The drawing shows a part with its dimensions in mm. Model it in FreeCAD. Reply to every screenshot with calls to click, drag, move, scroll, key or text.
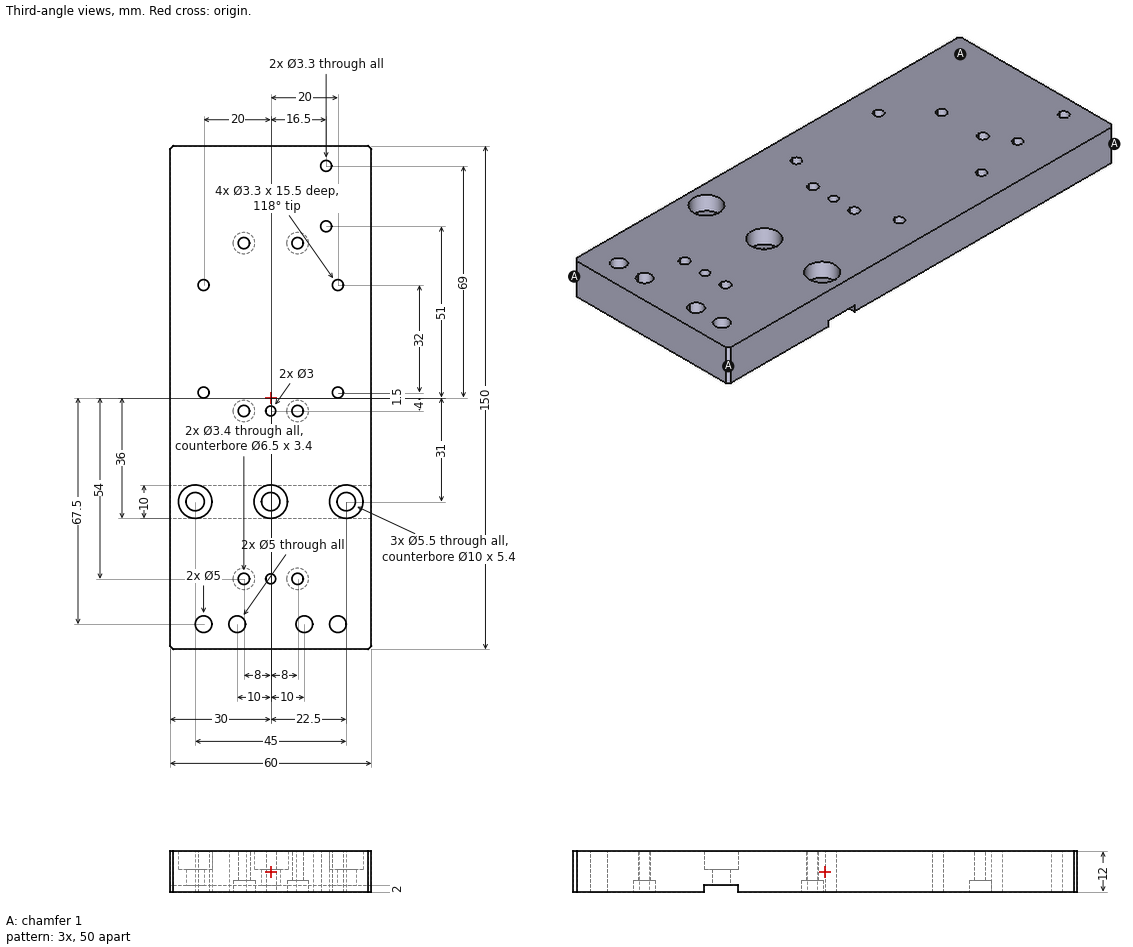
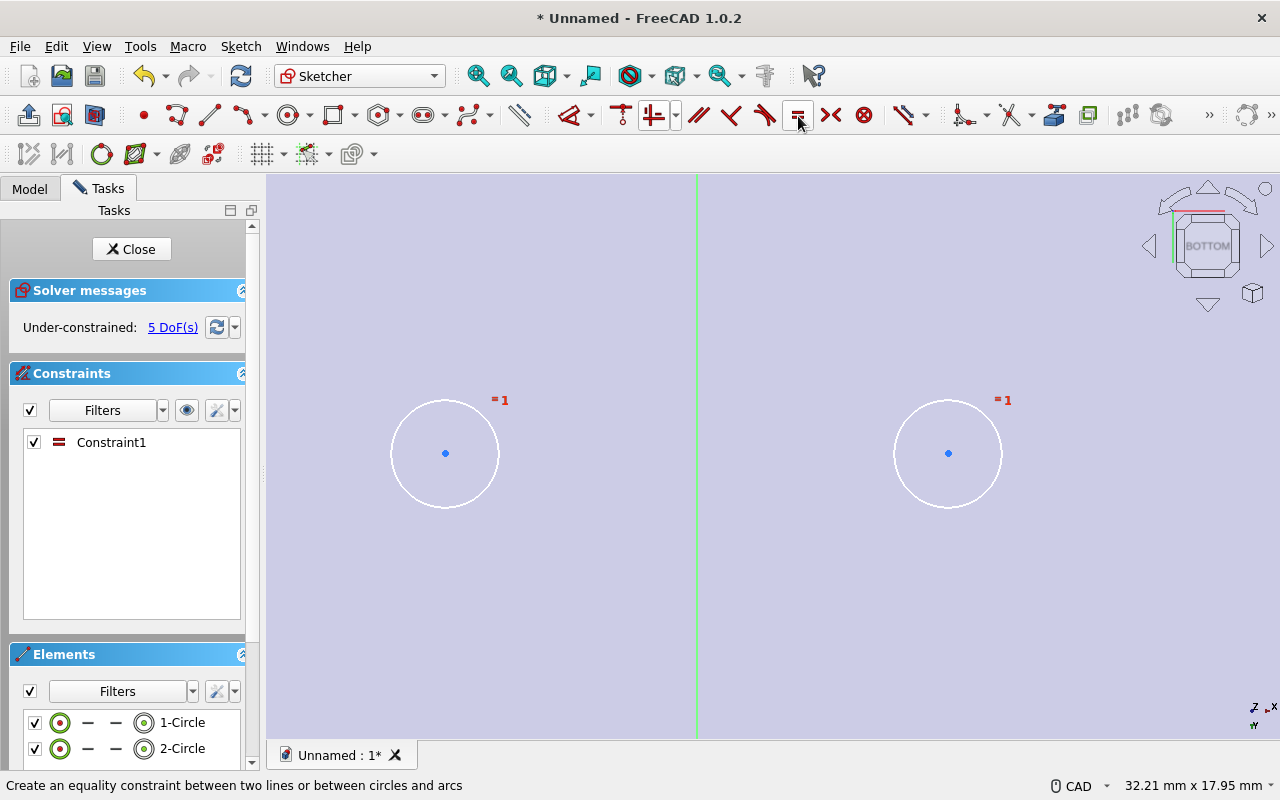
click(445, 454)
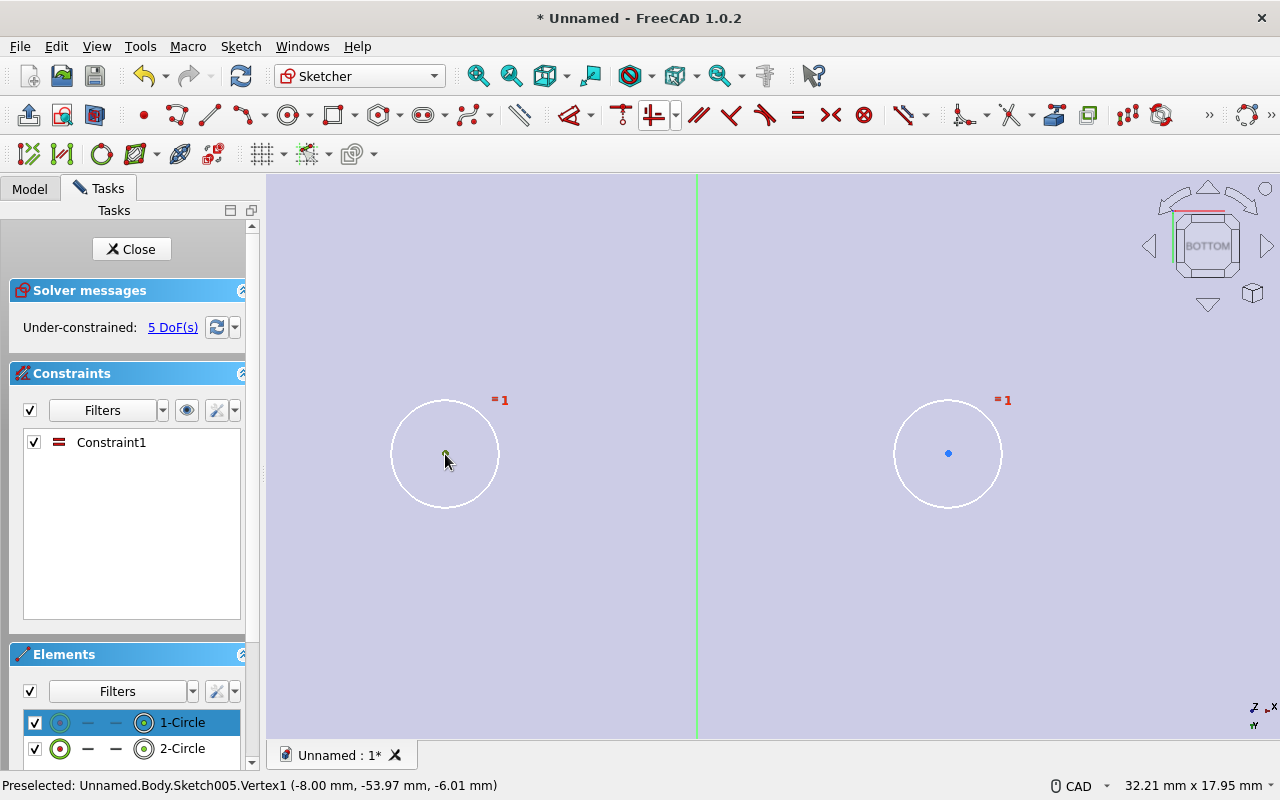
click(948, 454)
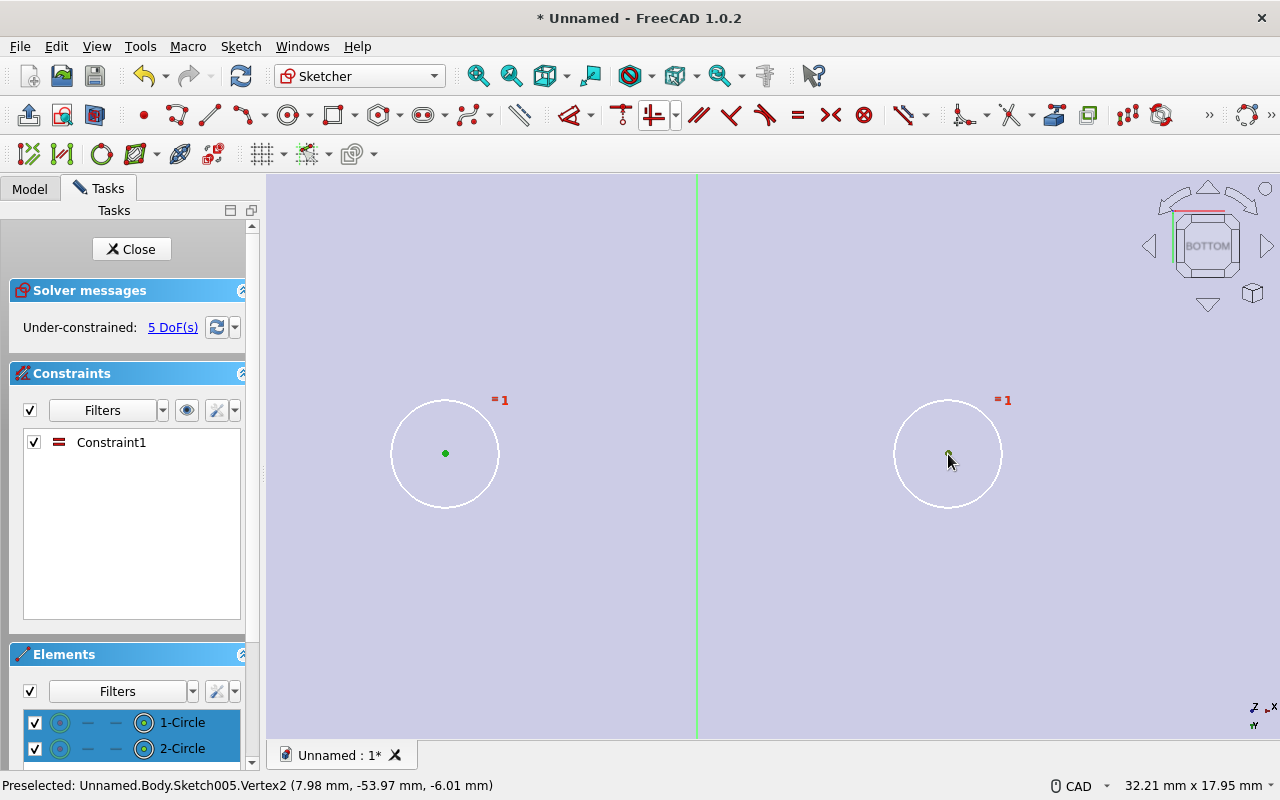
click(676, 116)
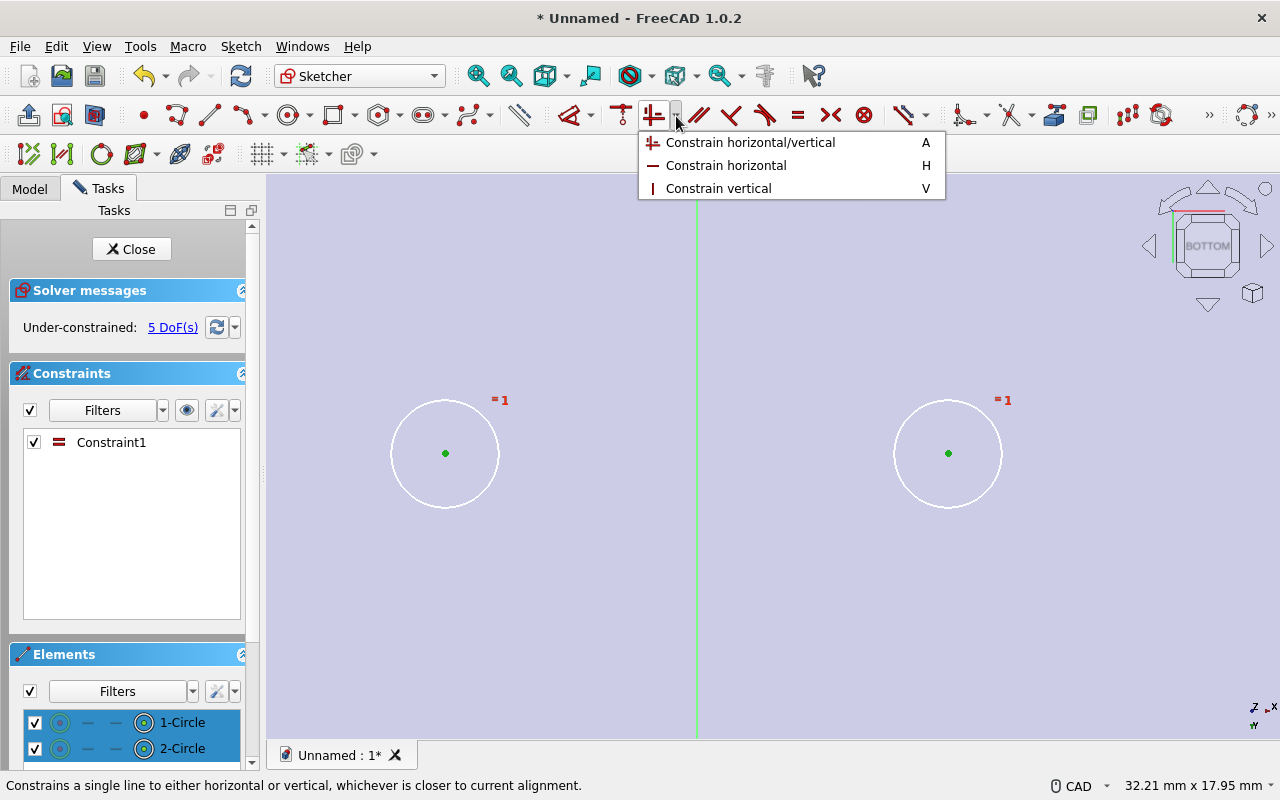
click(792, 166)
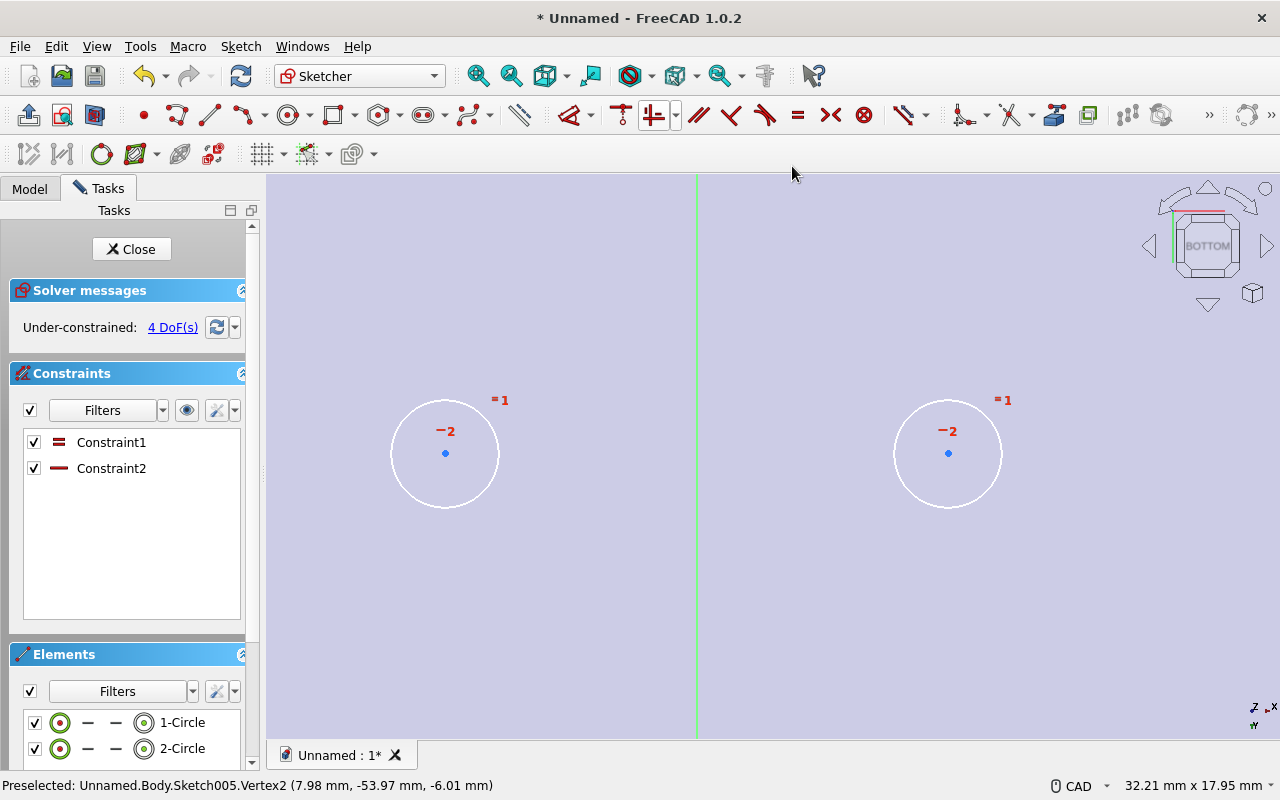
click(568, 116)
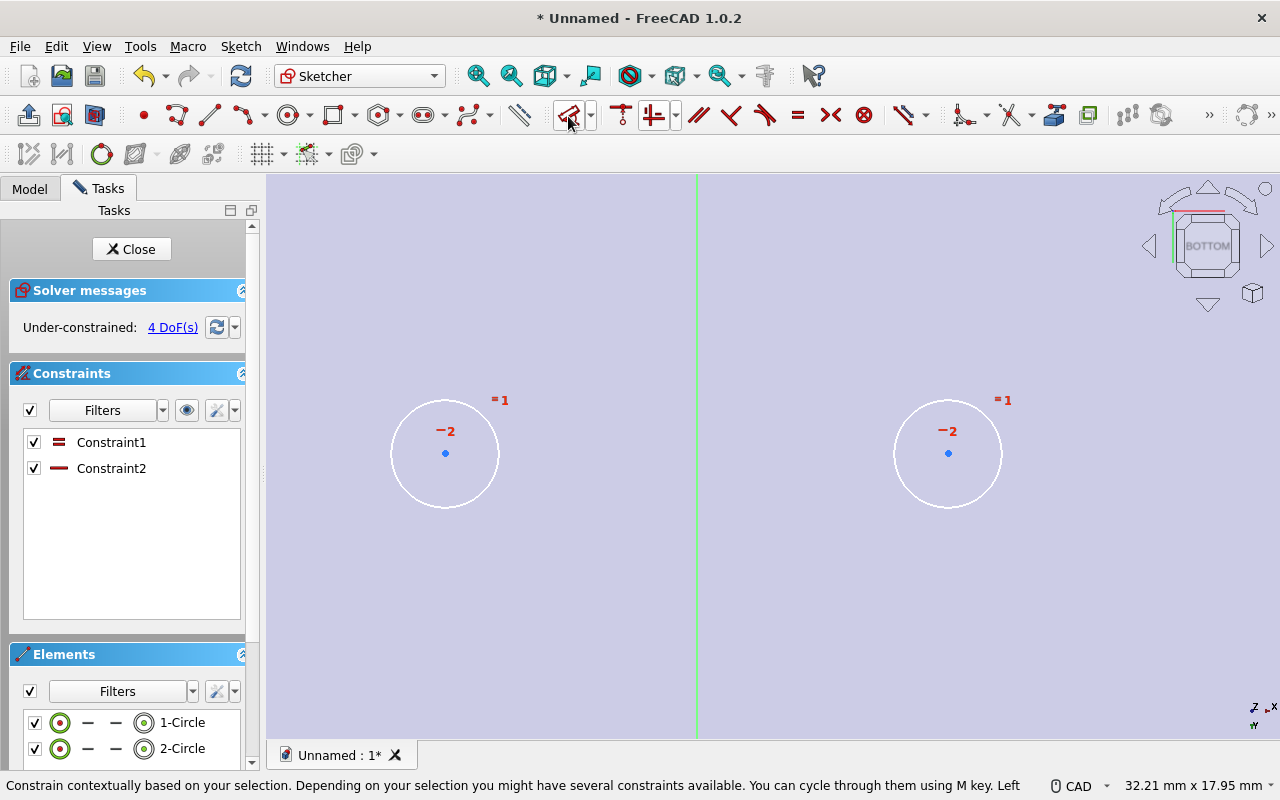
click(483, 416)
click(506, 393)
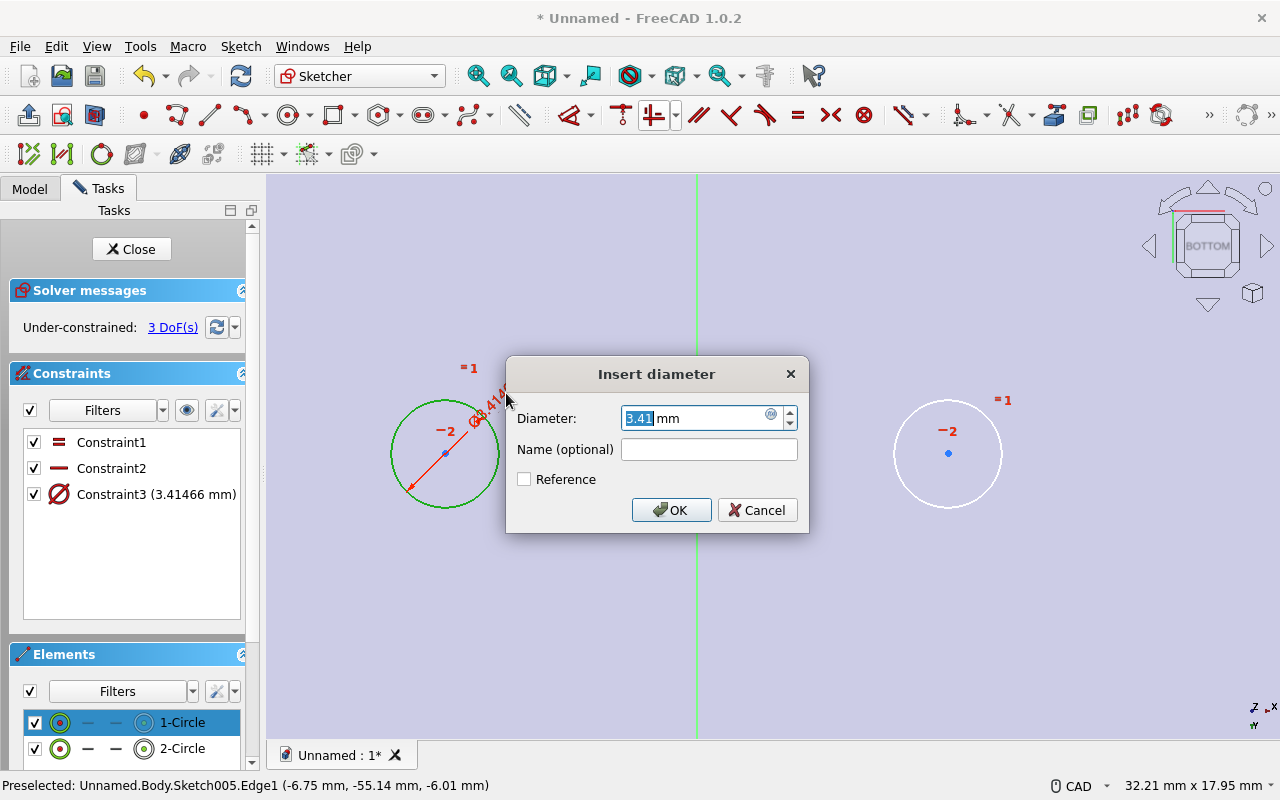
text(3.4)
key(Return)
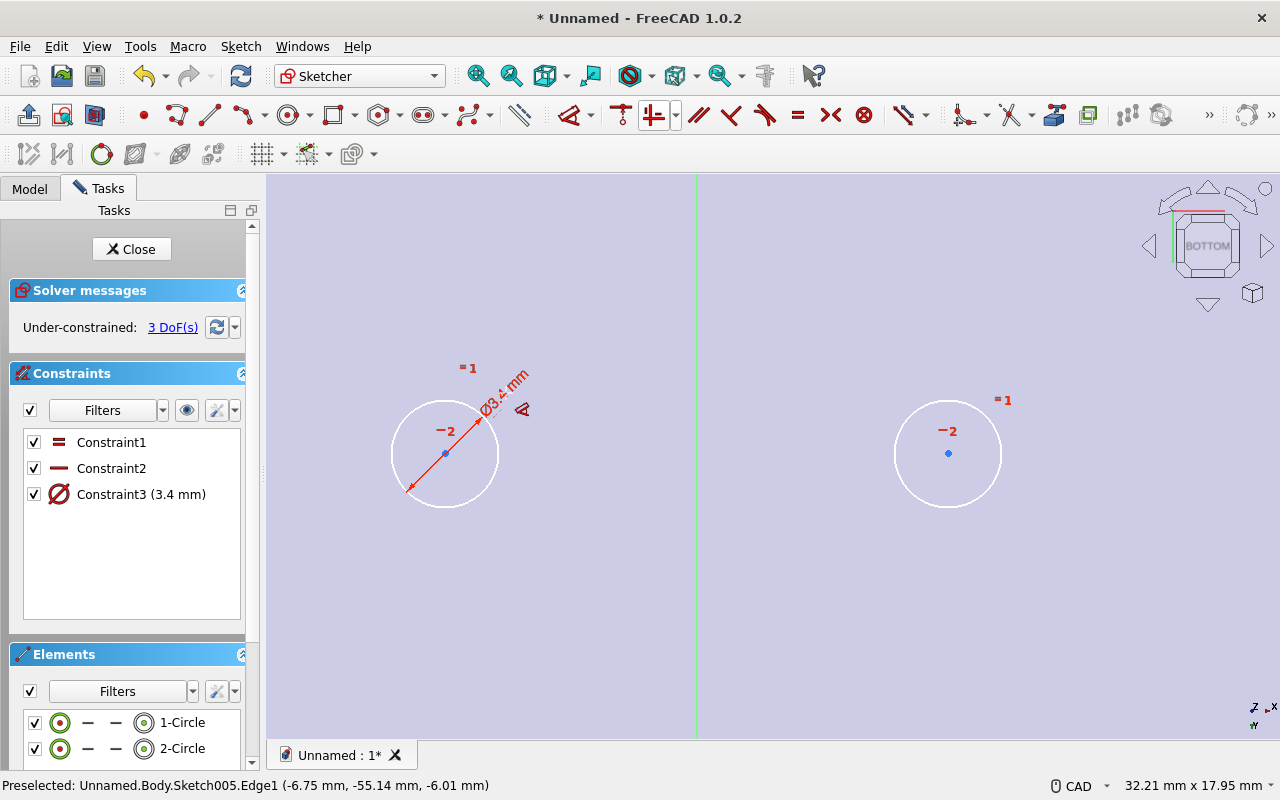
click(445, 454)
click(571, 420)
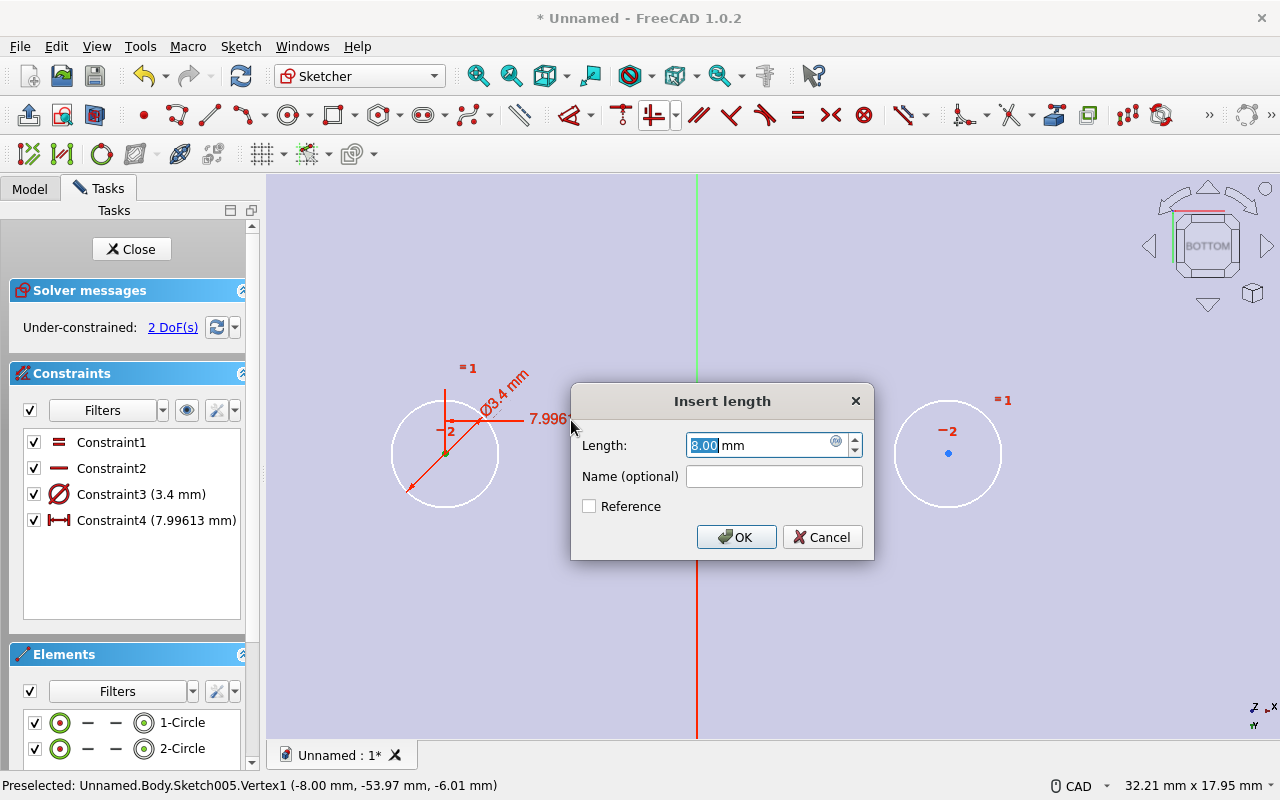
text(8)
key(Return)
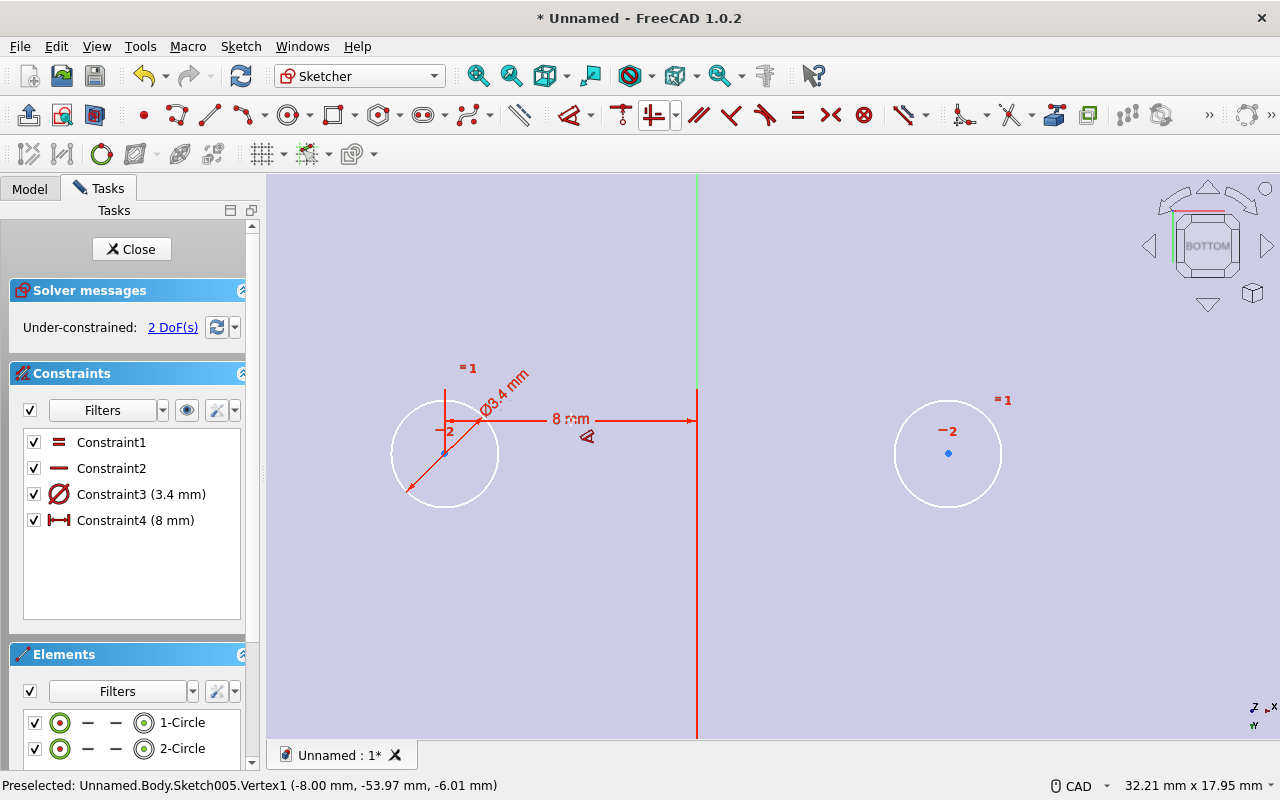
click(948, 454)
click(822, 420)